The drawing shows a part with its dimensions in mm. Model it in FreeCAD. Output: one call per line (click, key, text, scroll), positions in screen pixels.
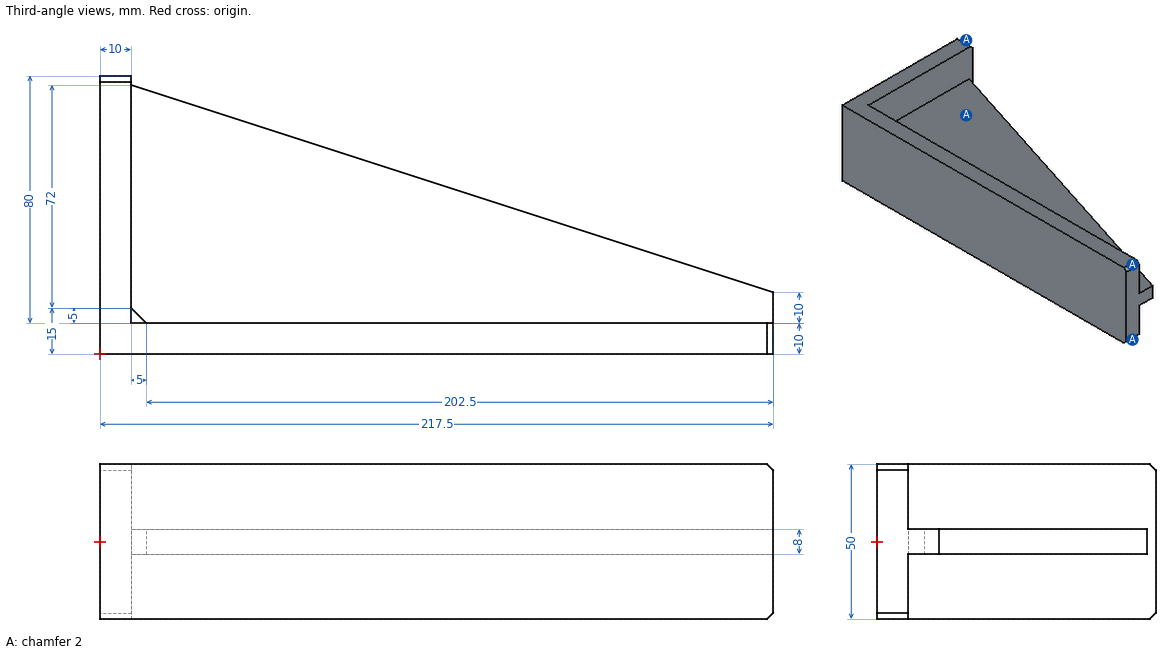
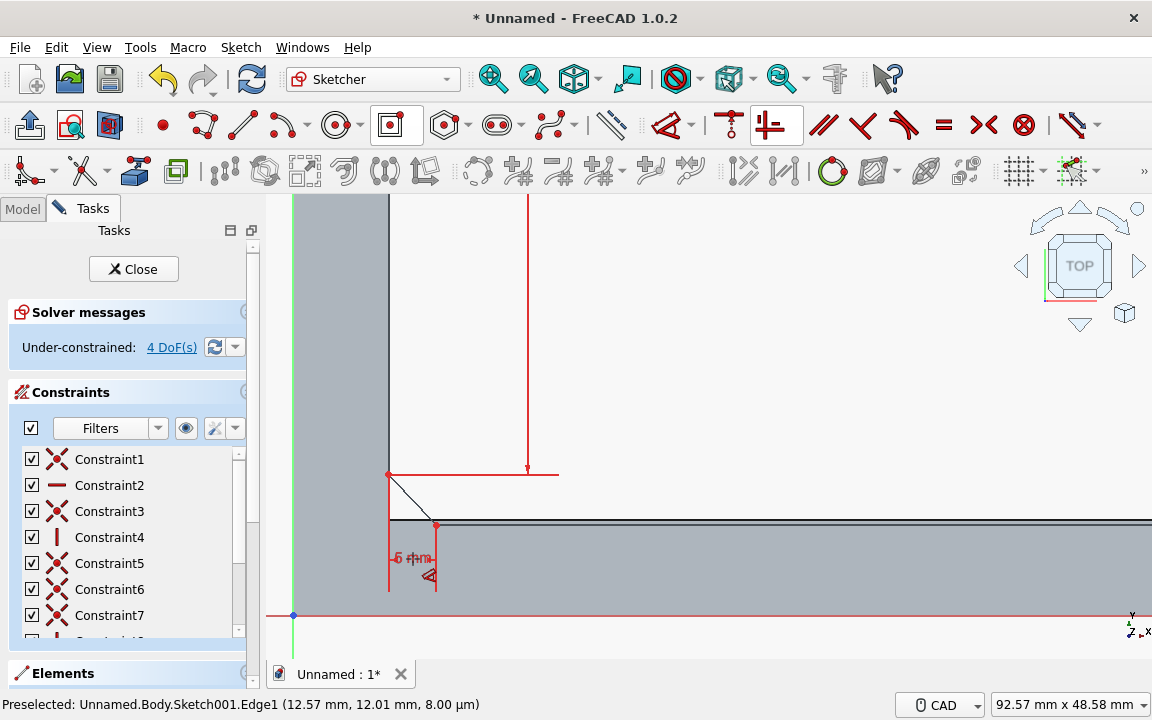
click(403, 490)
click(355, 500)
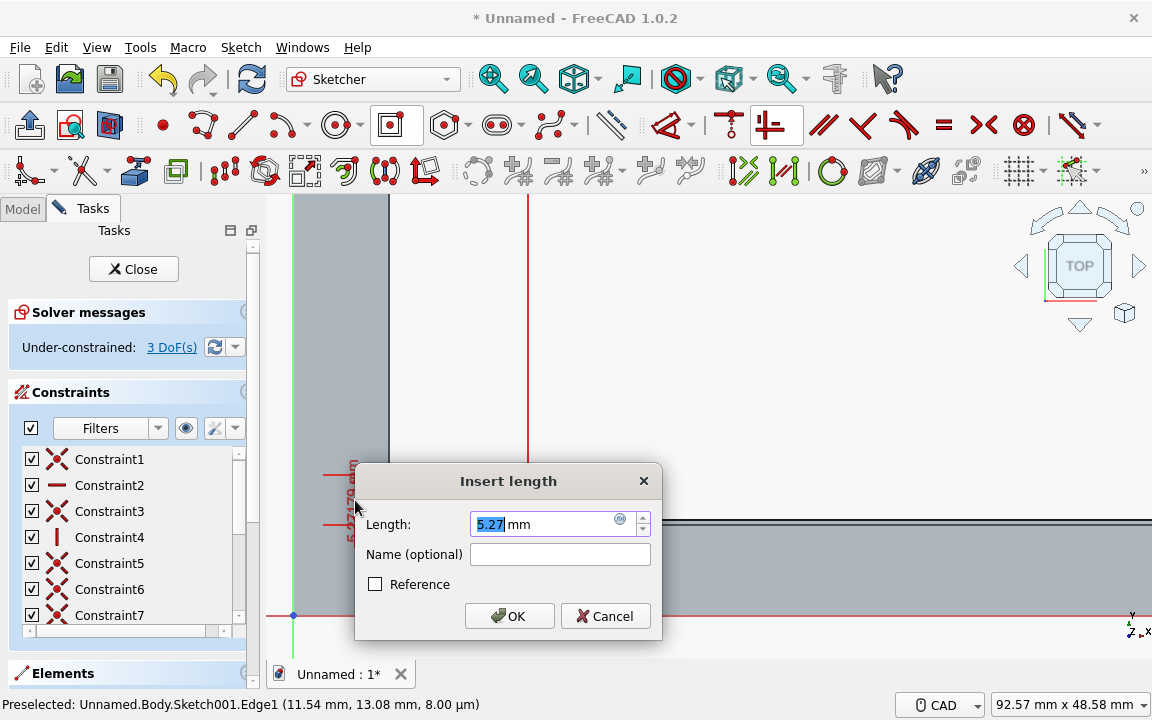
text(5)
key(Return)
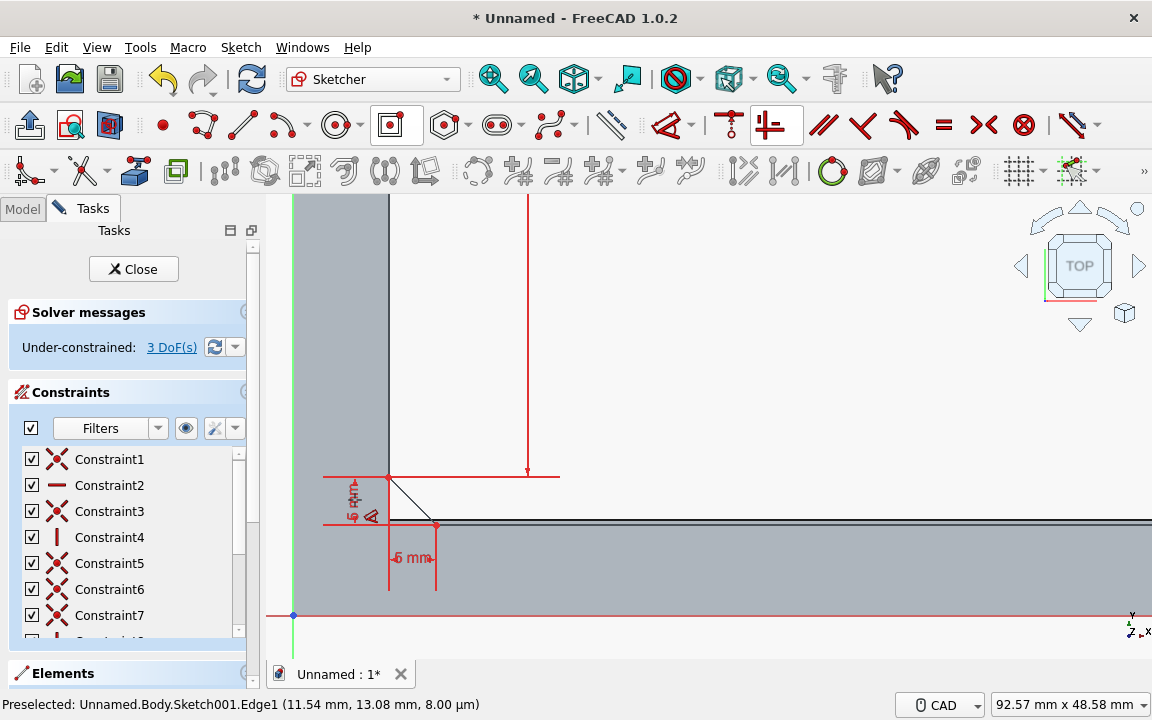
click(389, 477)
click(341, 443)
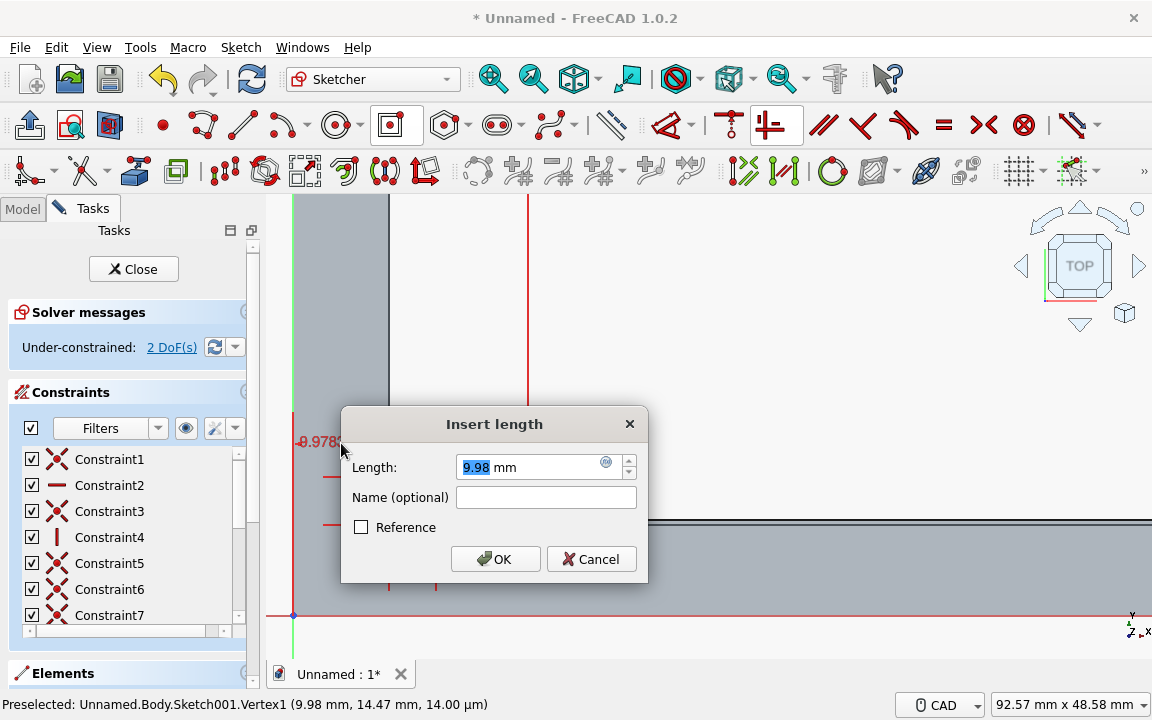
text(10)
key(Return)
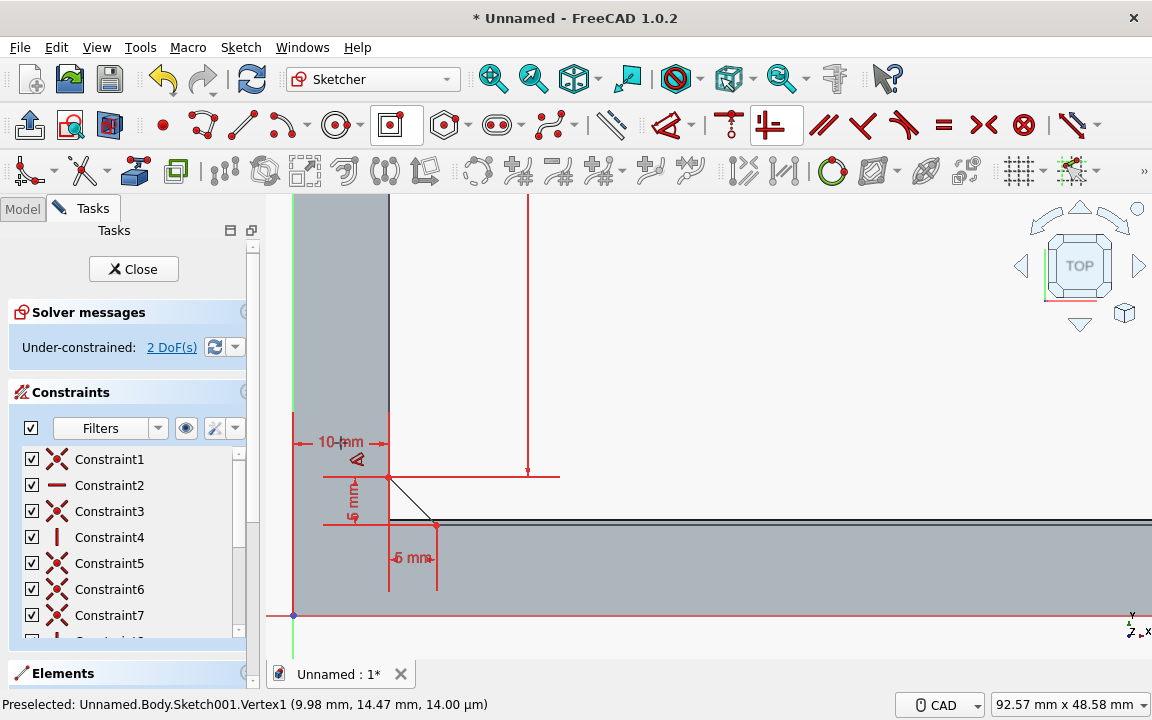
scroll(414, 501, down, 7)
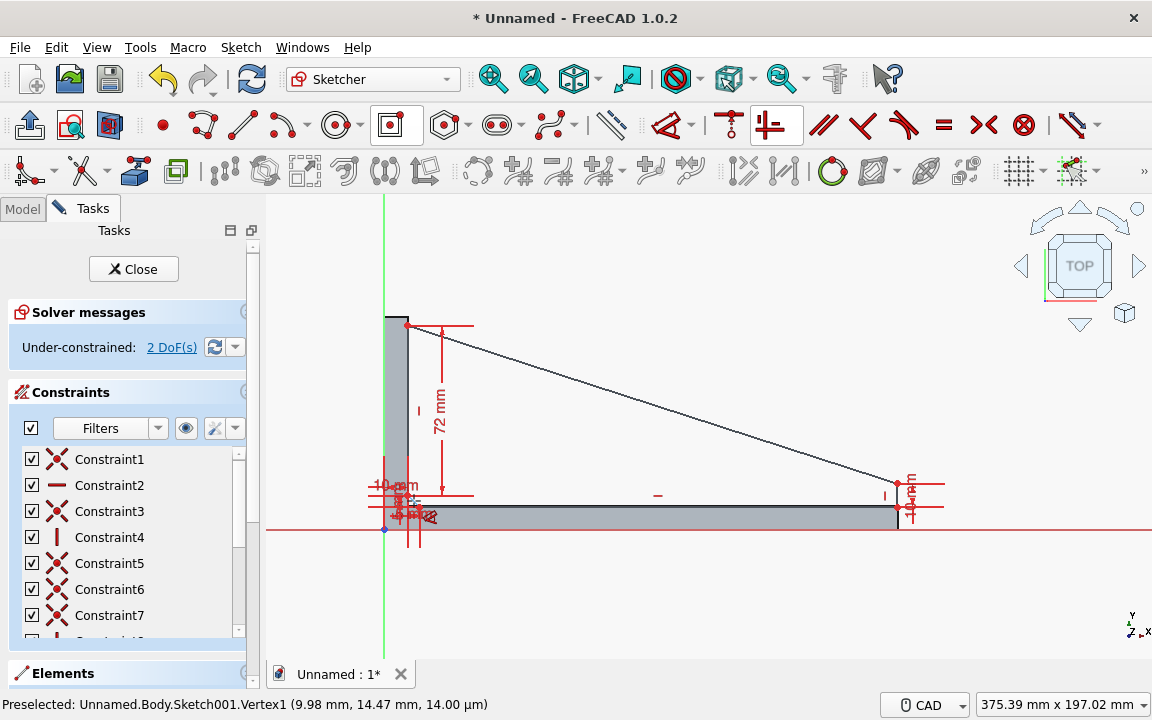
click(408, 496)
click(326, 513)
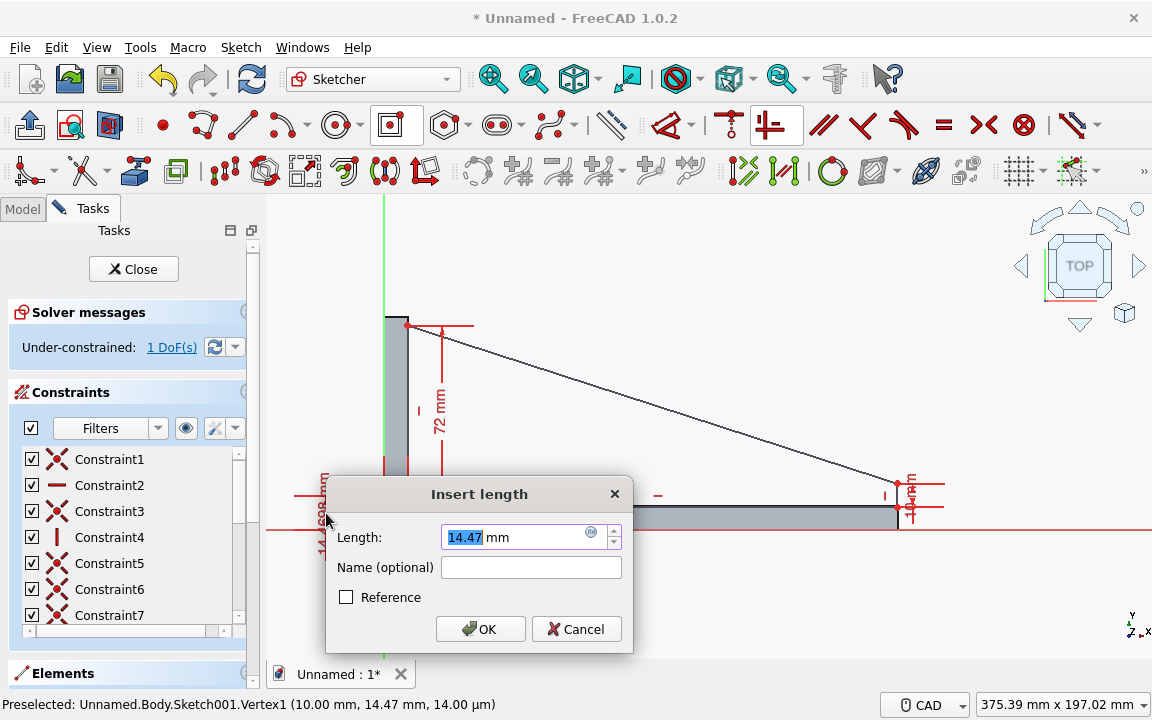
text(15)
key(Return)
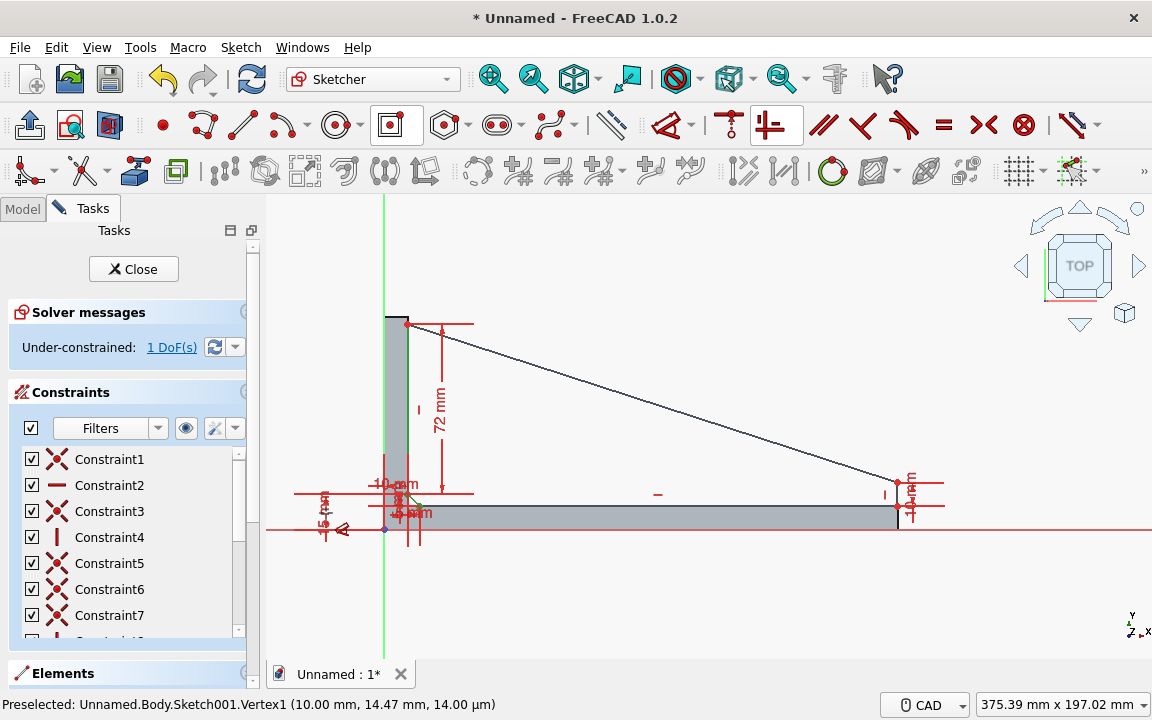
click(563, 506)
click(659, 472)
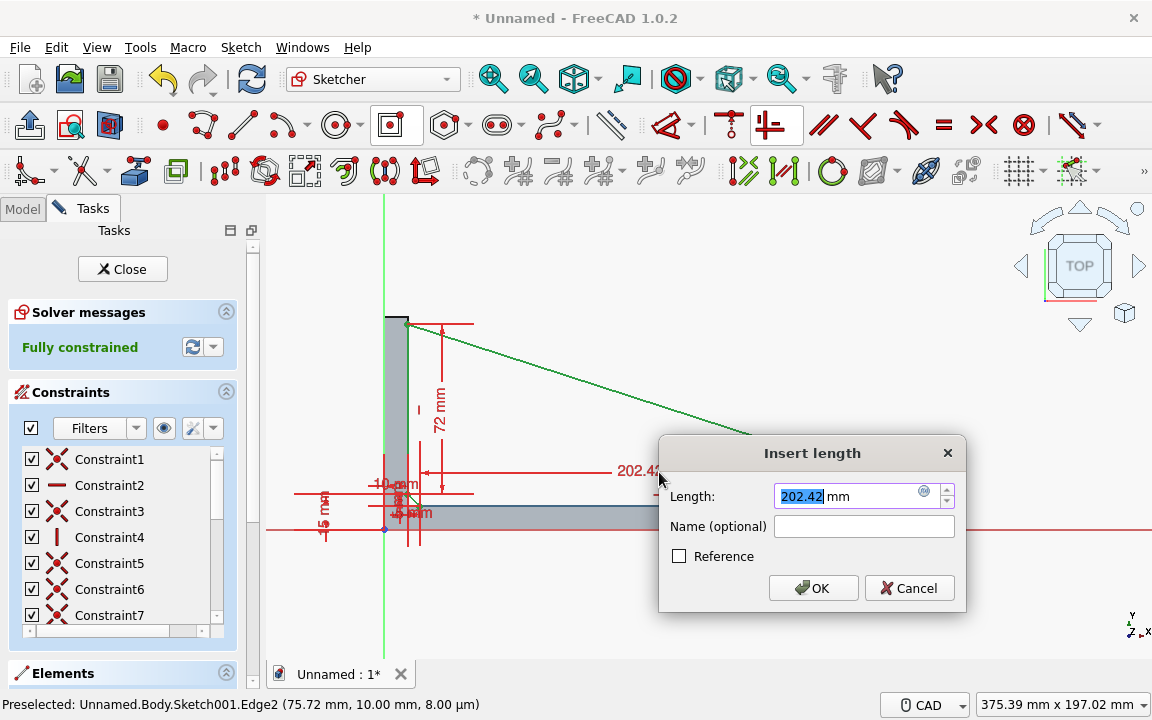
text(202.5)
key(Return)
key(Escape)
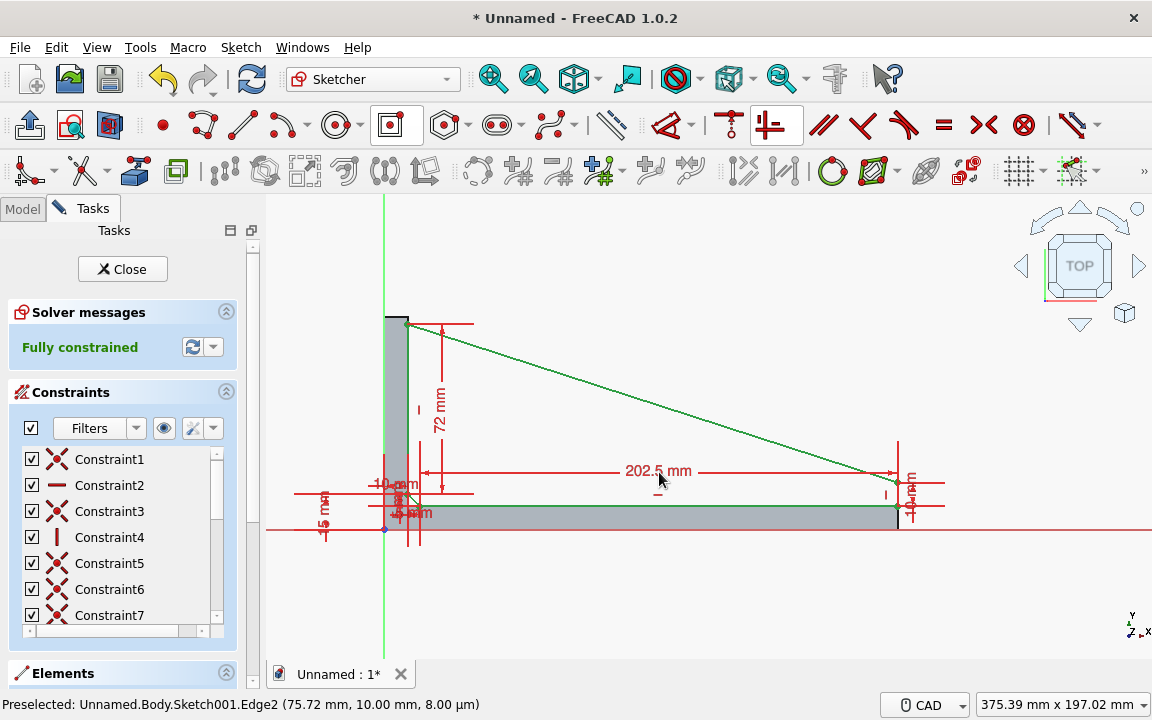
click(123, 269)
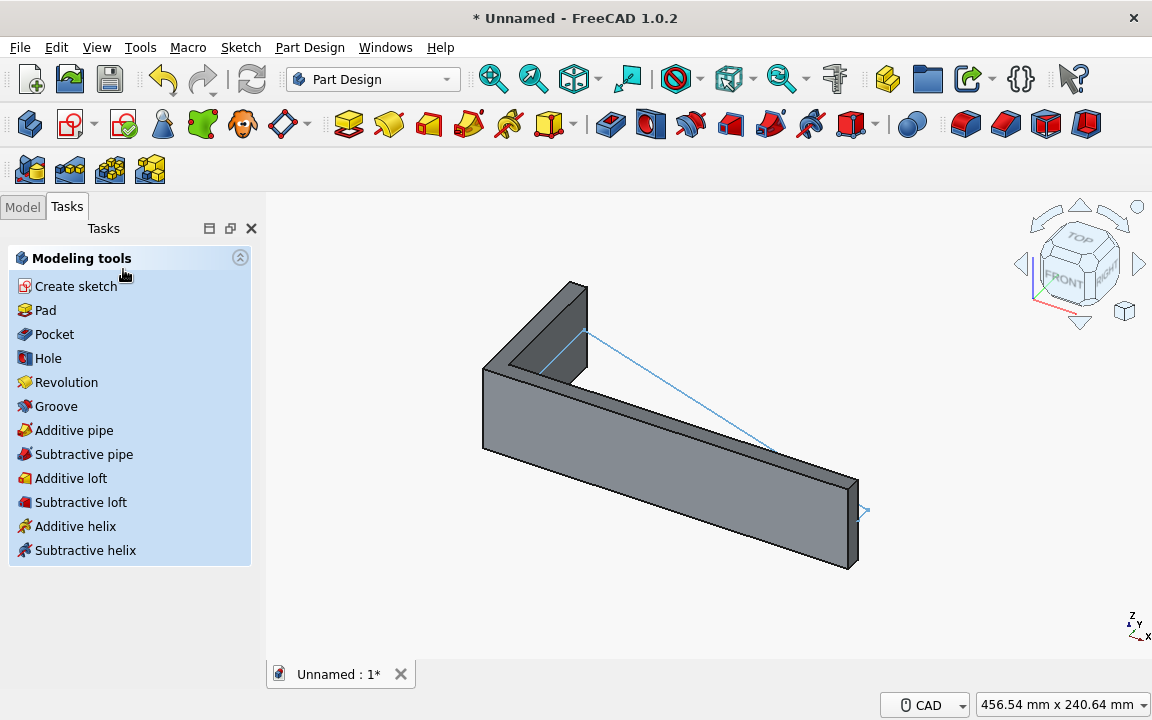
click(350, 124)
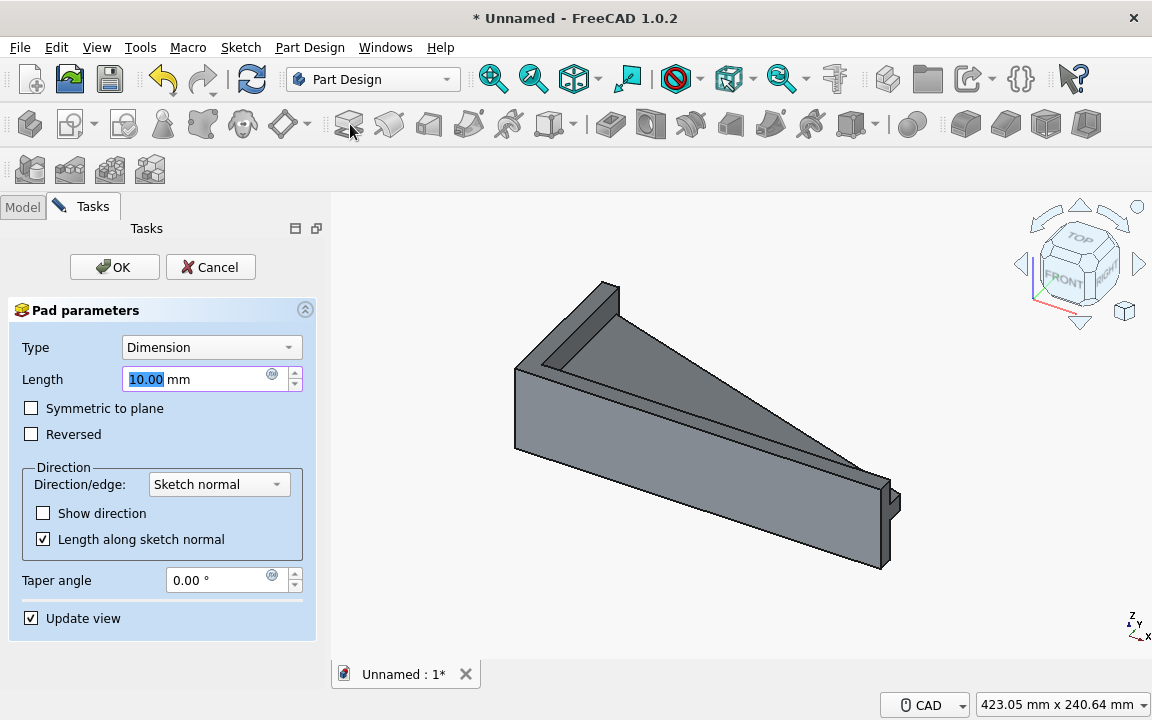
text(8)
key(Tab)